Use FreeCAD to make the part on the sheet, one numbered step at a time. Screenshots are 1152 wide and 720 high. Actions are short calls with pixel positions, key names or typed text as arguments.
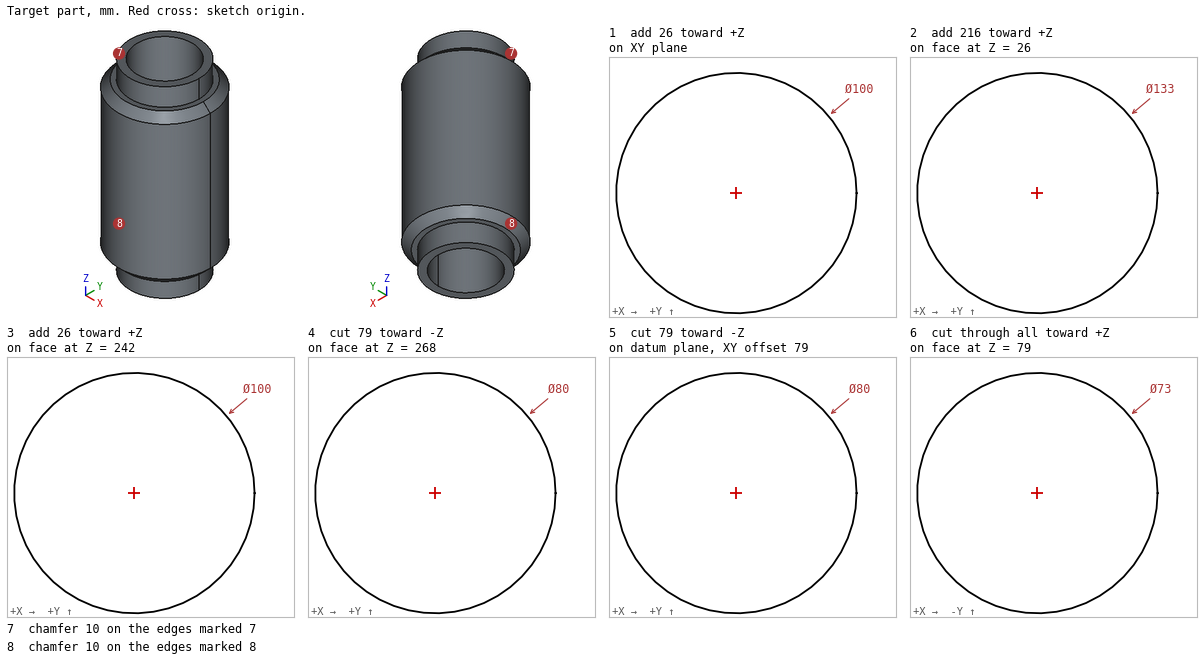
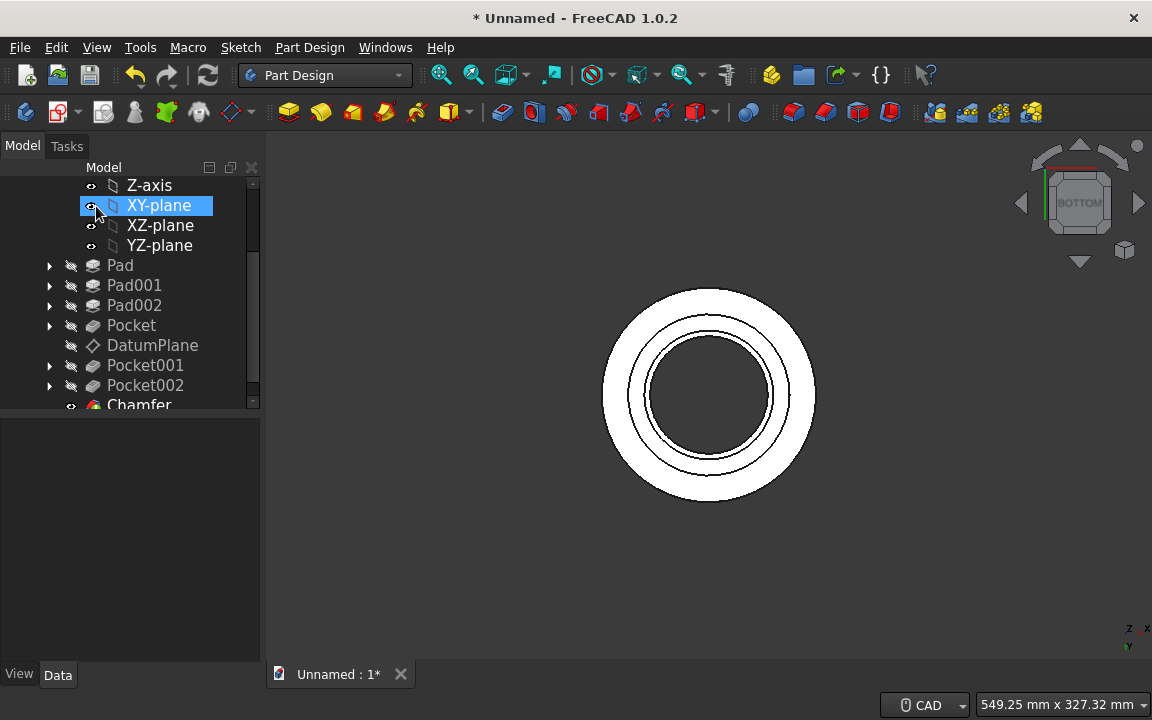
key(v)
key(f)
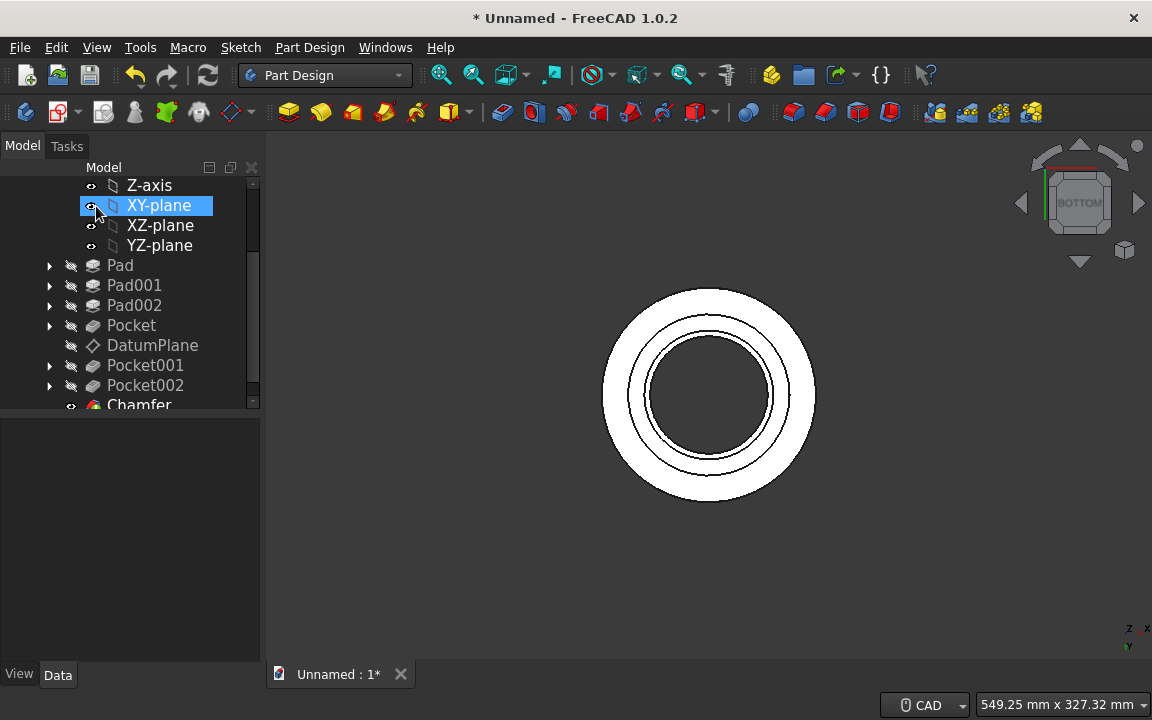
click(602, 394)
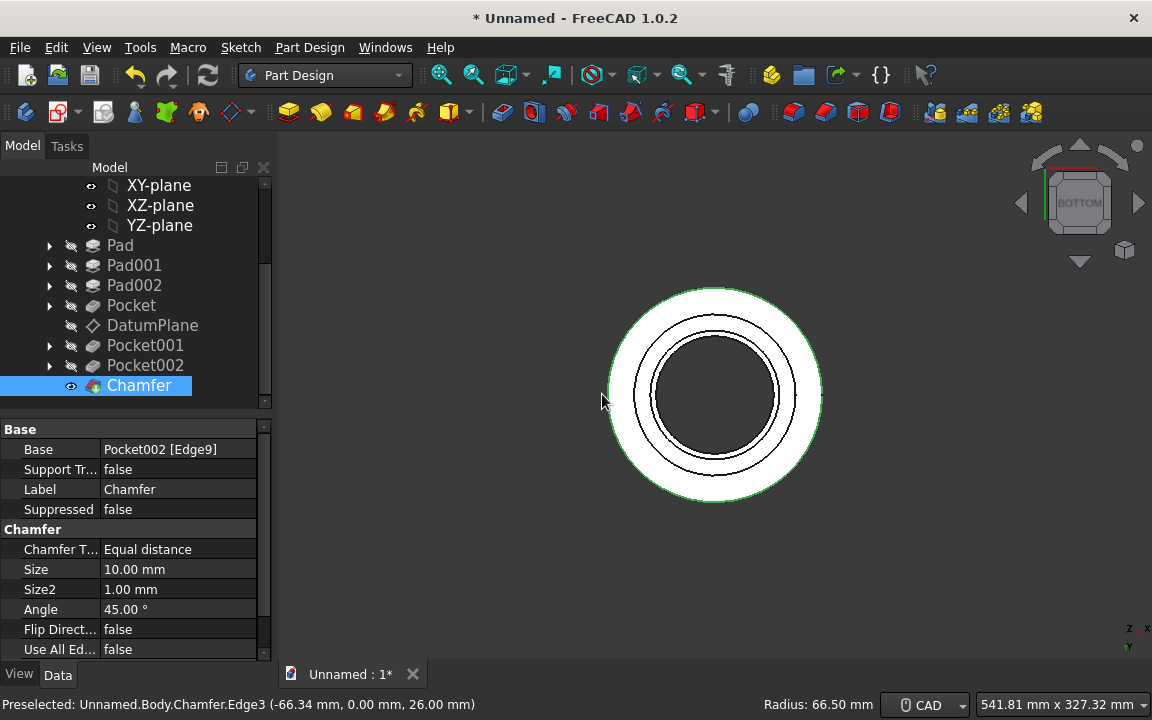
click(826, 112)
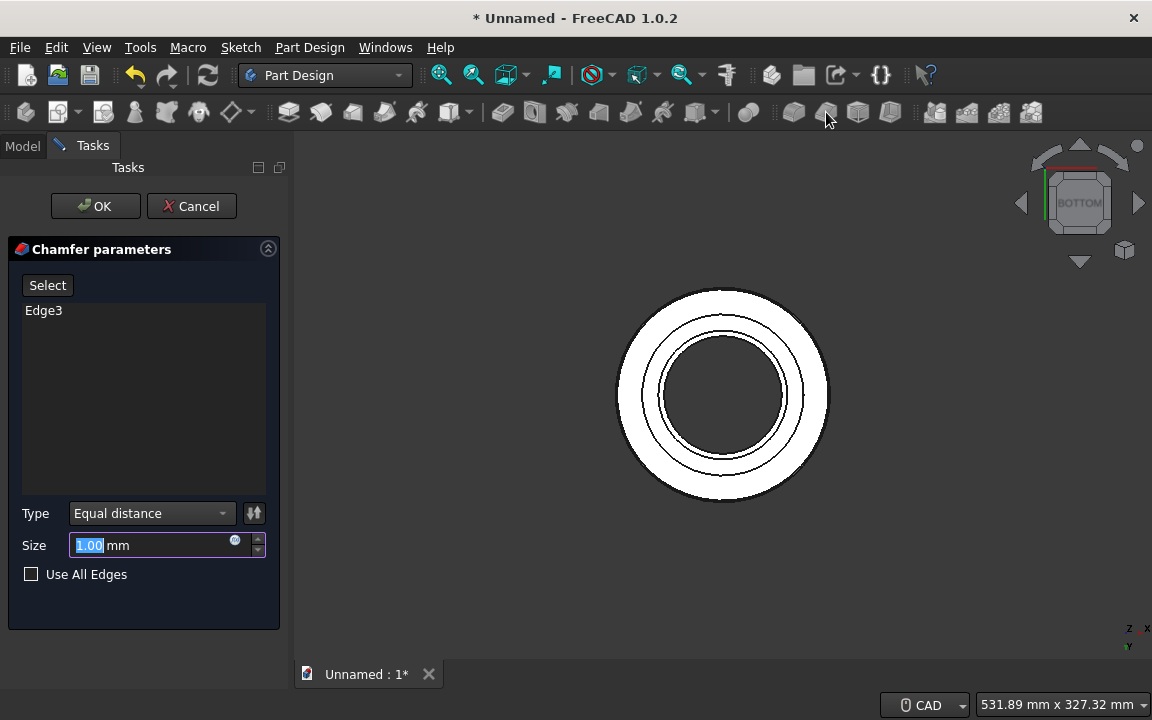
text(10)
key(Tab)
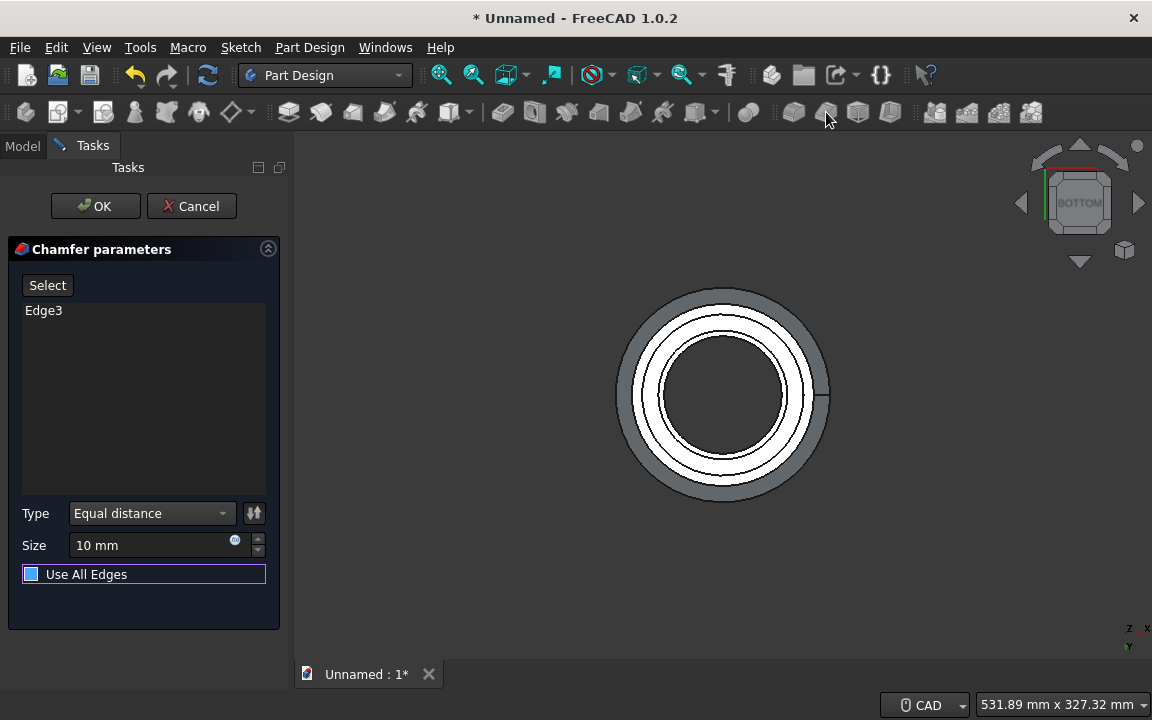
click(96, 206)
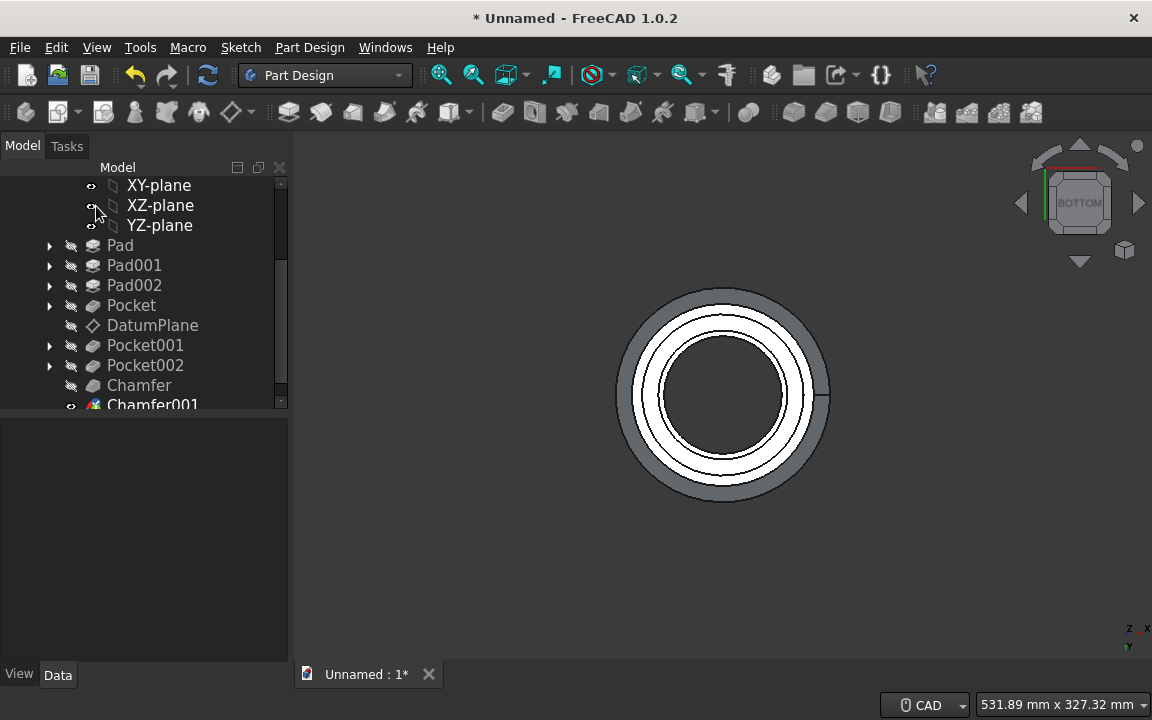
key(0)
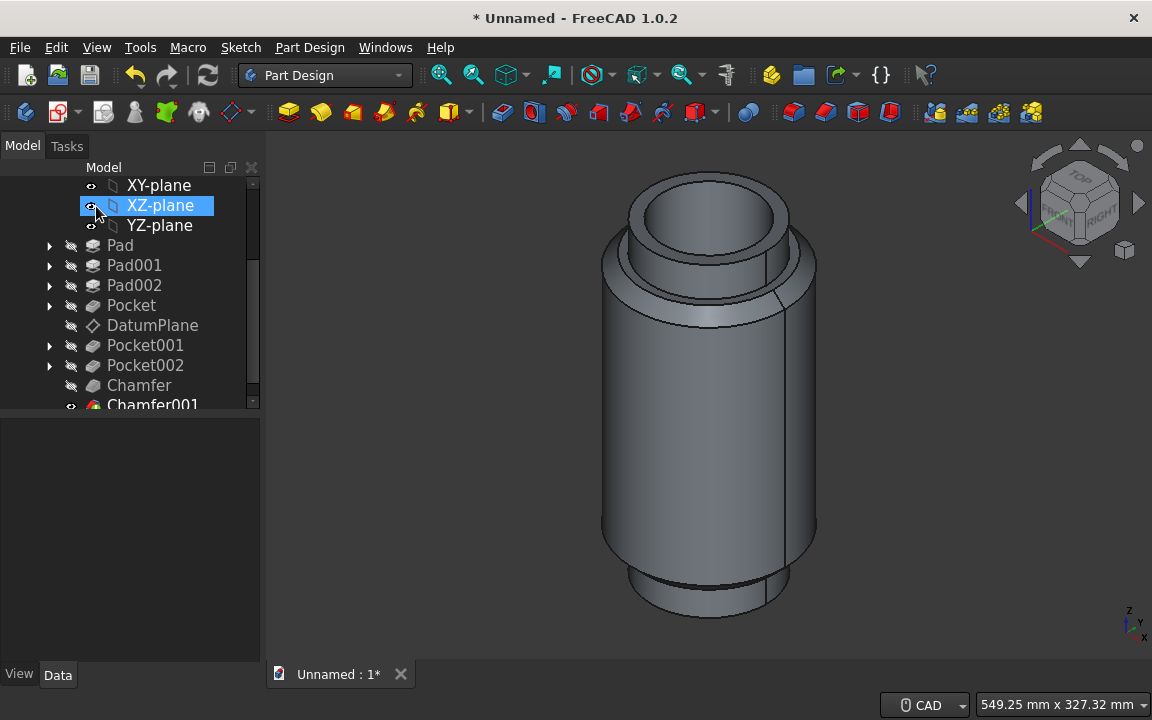
key(v)
key(f)